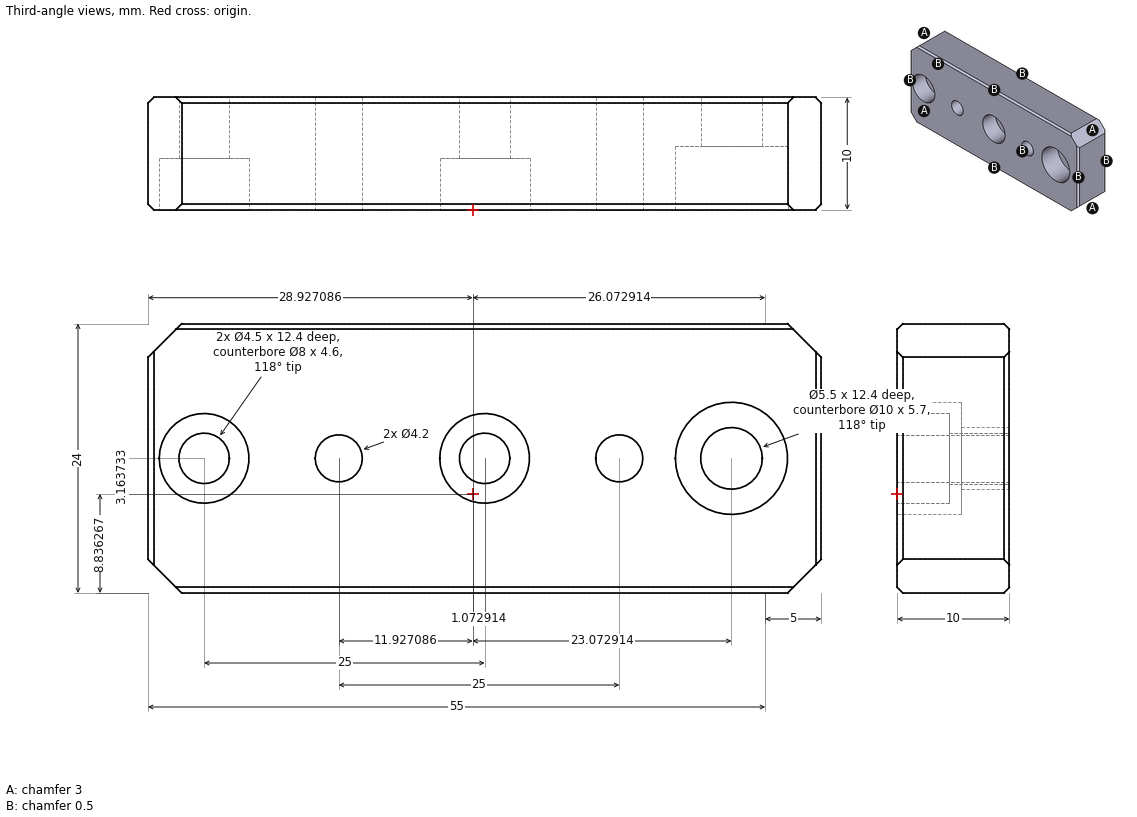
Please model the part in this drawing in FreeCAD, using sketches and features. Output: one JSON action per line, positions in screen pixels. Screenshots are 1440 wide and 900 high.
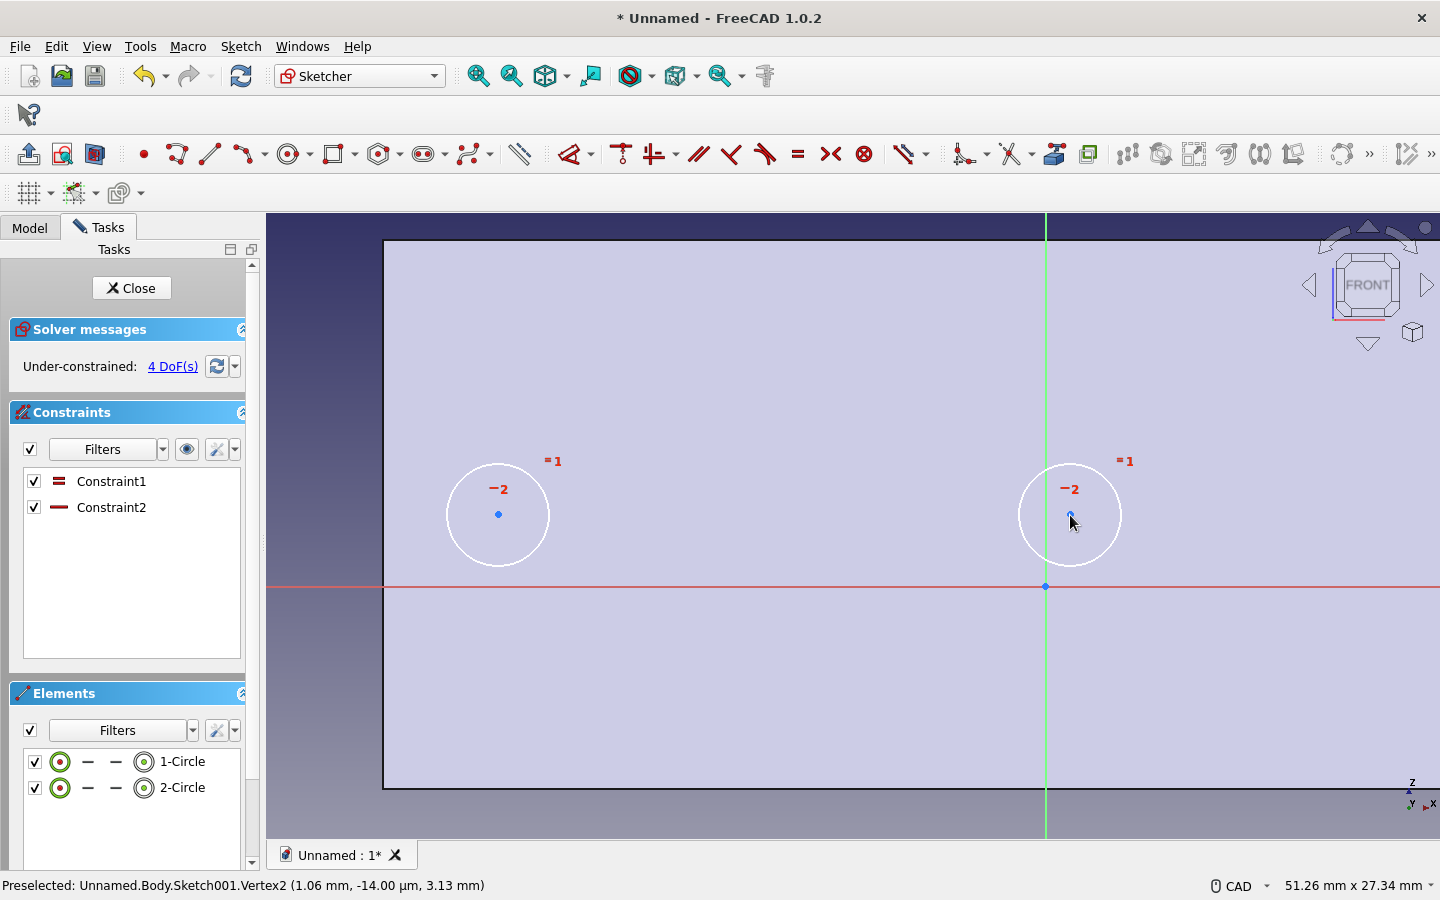
{"action": "left_click", "coordinate": [568, 154]}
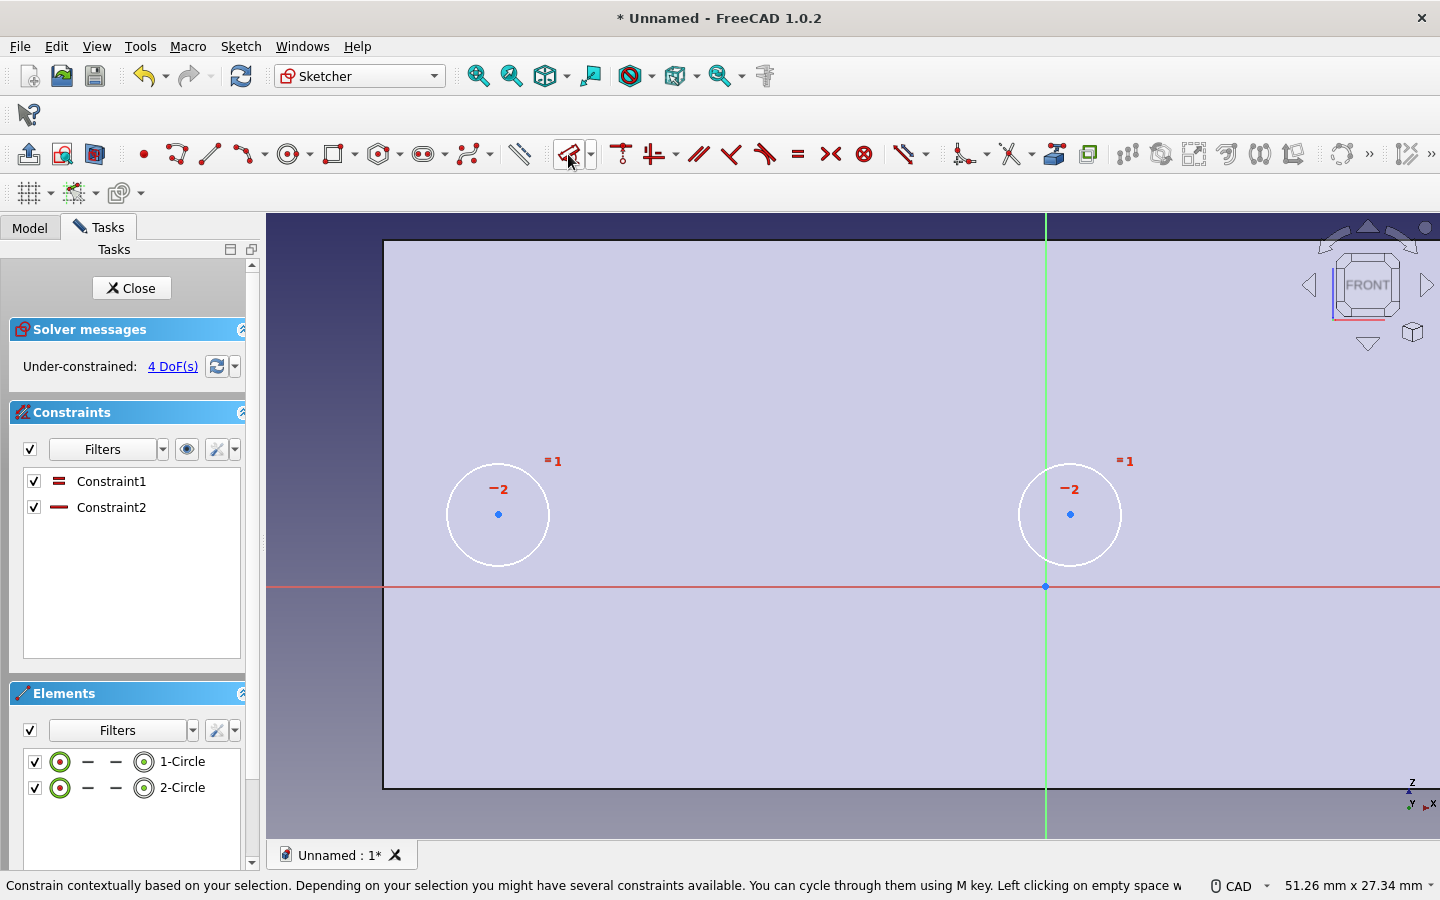
{"action": "left_click", "coordinate": [534, 479]}
{"action": "left_click", "coordinate": [557, 456]}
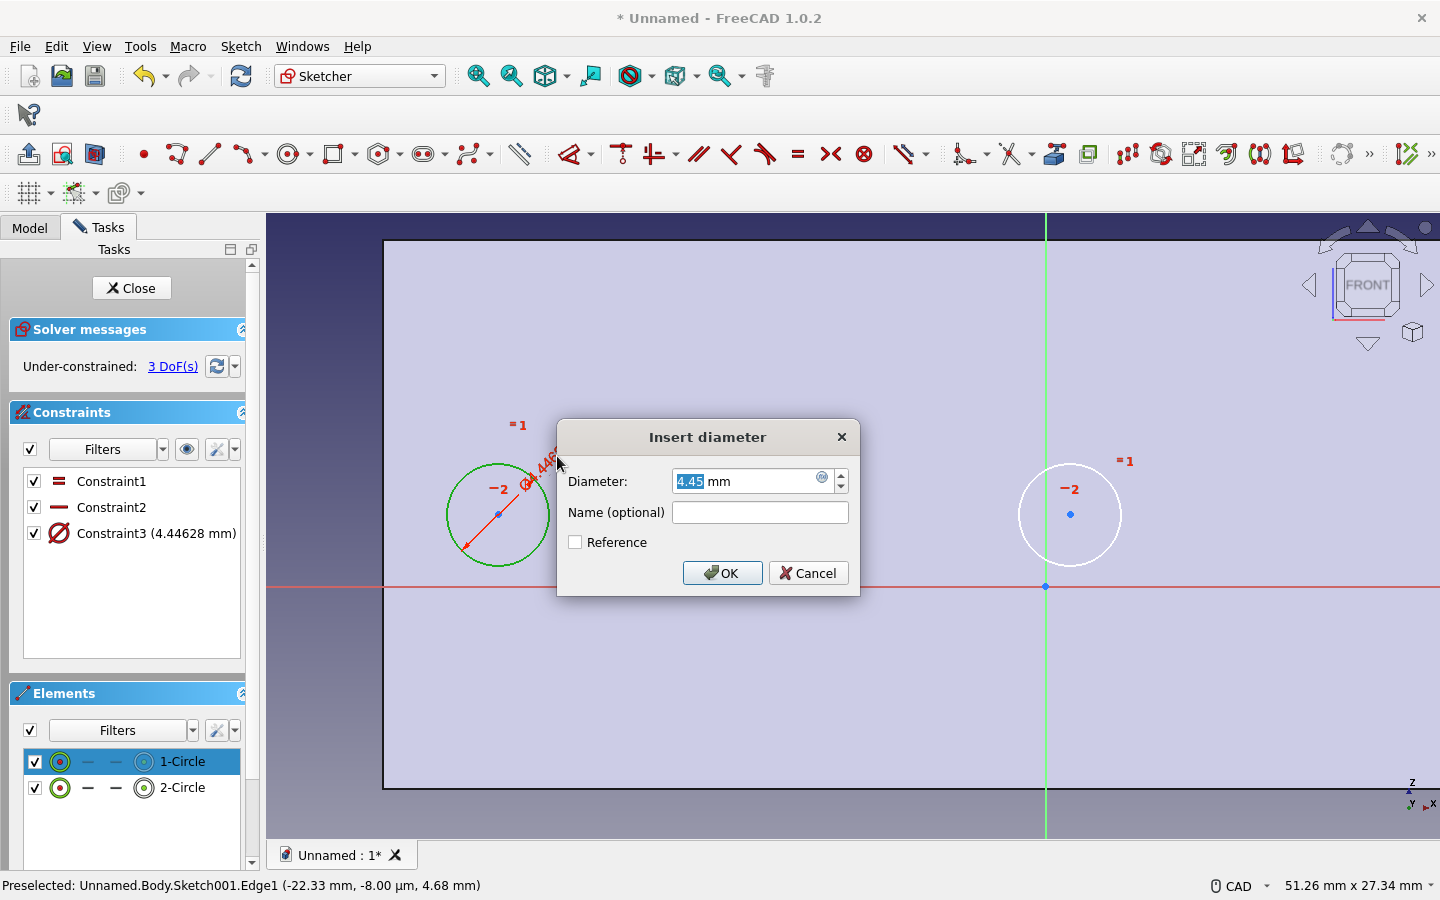
{"action": "type", "text": "4.5"}
{"action": "key", "text": "Return"}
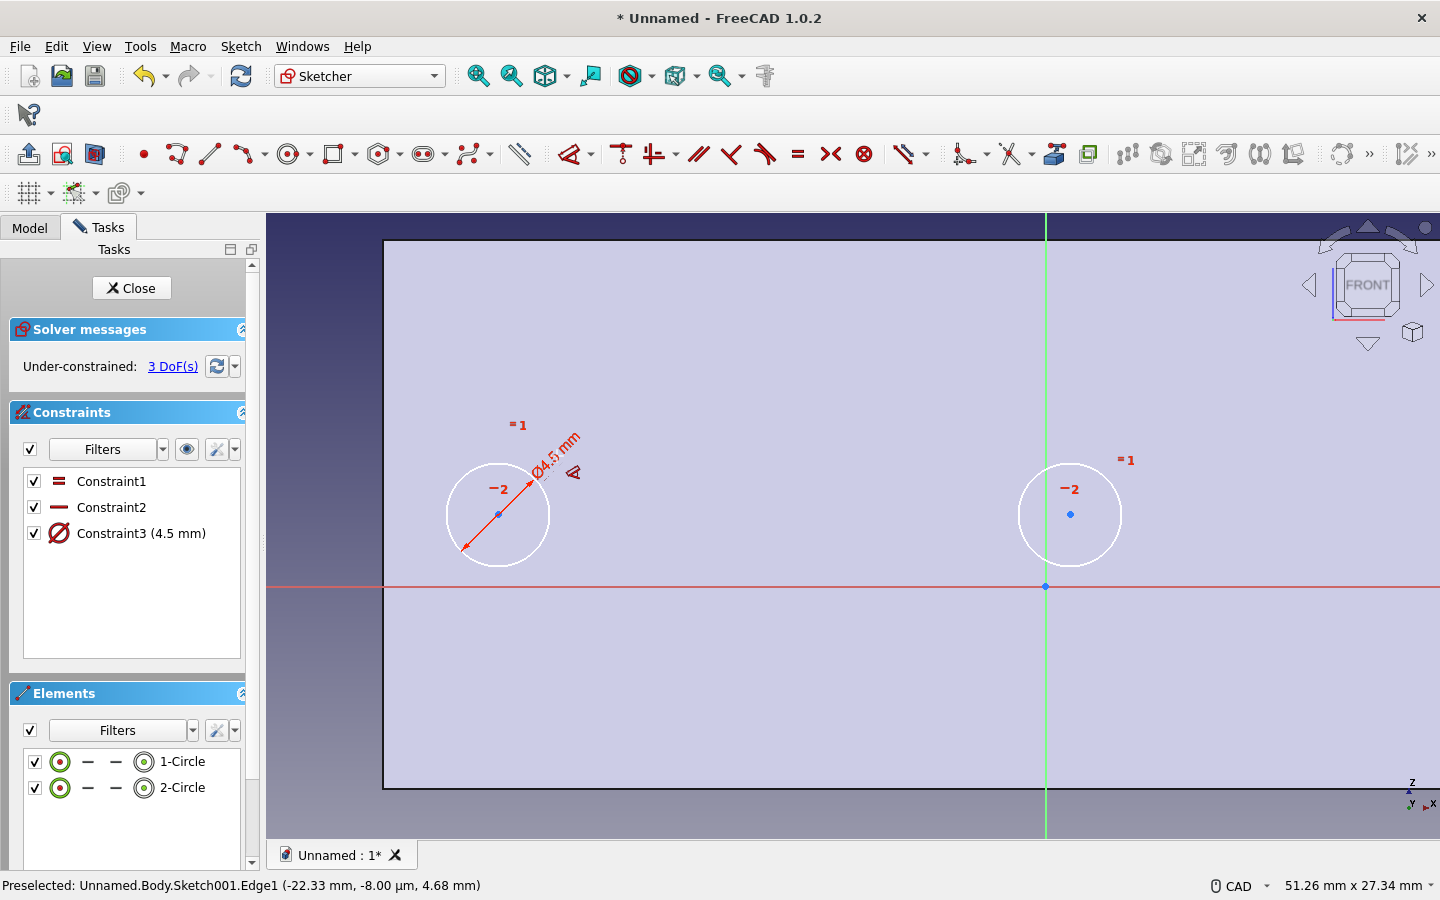
{"action": "left_click", "coordinate": [498, 515]}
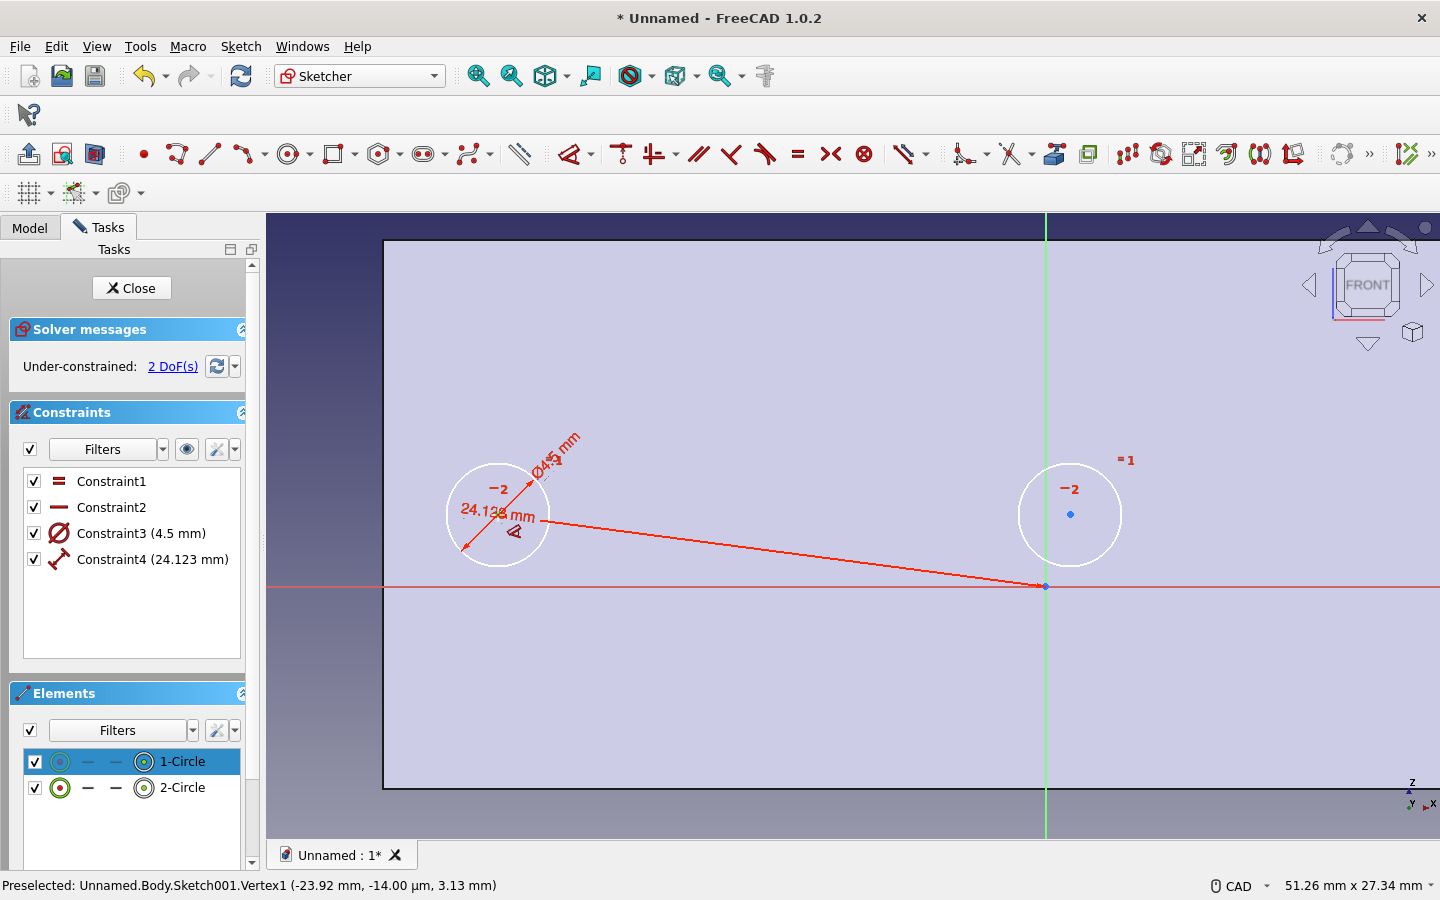
{"action": "left_click", "coordinate": [1070, 515]}
{"action": "left_click", "coordinate": [784, 481]}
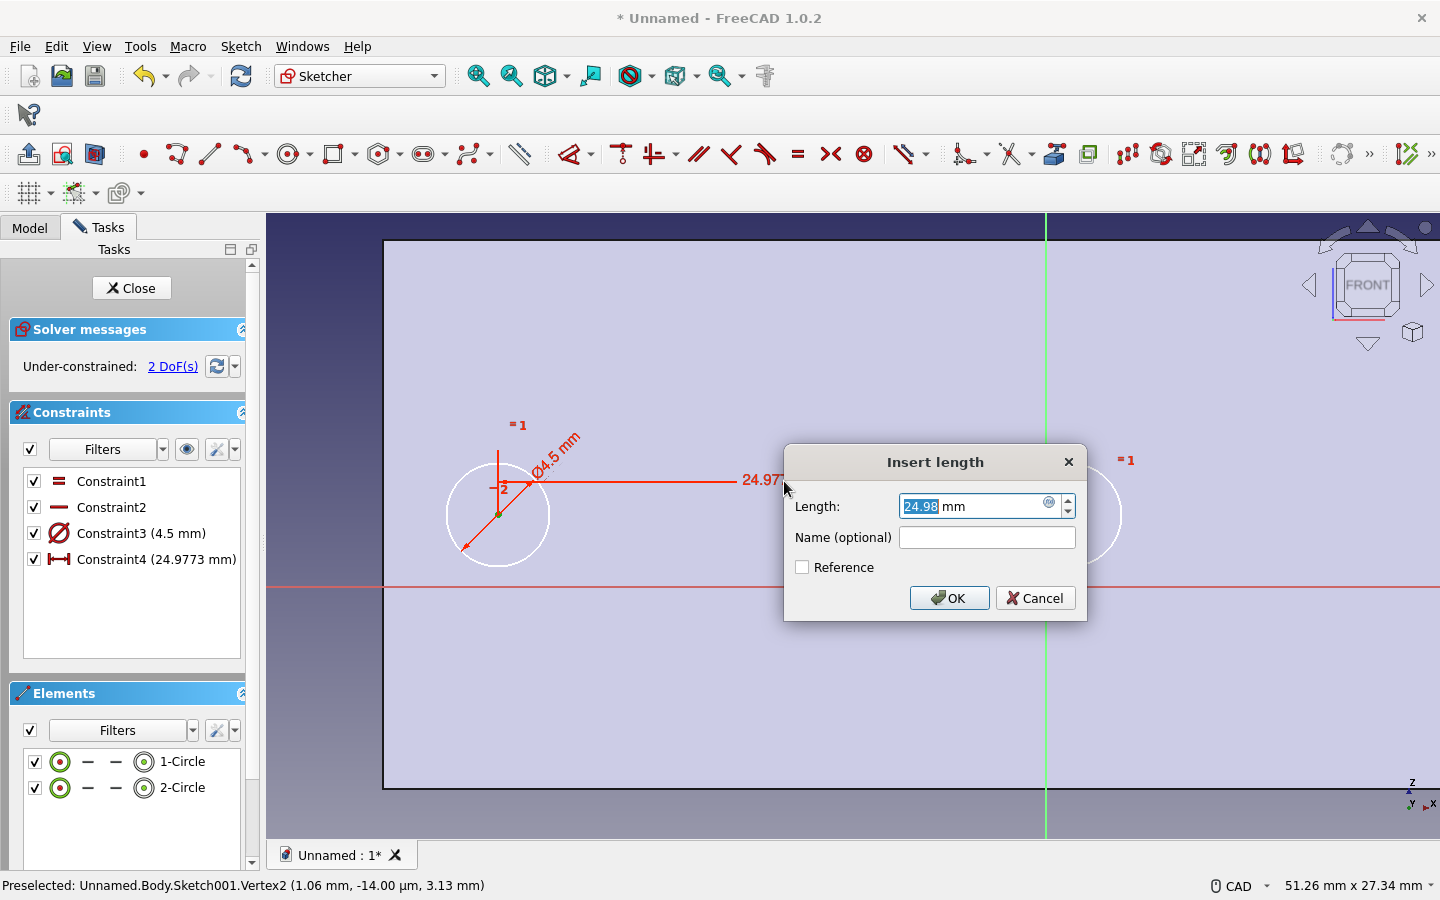
{"action": "type", "text": "25"}
{"action": "key", "text": "Return"}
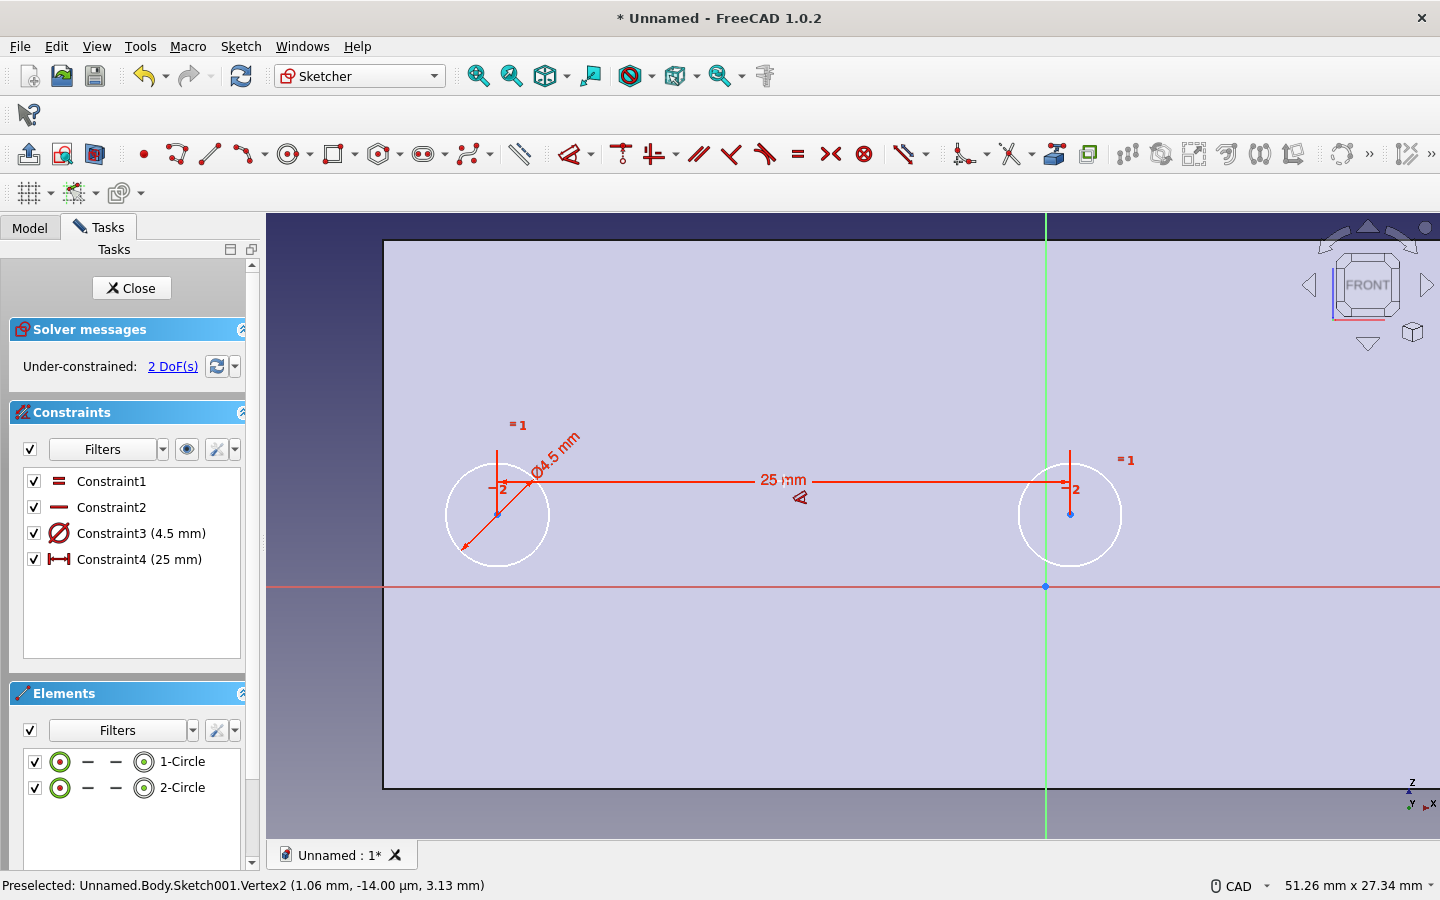
{"action": "left_click", "coordinate": [497, 515]}
{"action": "left_click", "coordinate": [463, 526]}